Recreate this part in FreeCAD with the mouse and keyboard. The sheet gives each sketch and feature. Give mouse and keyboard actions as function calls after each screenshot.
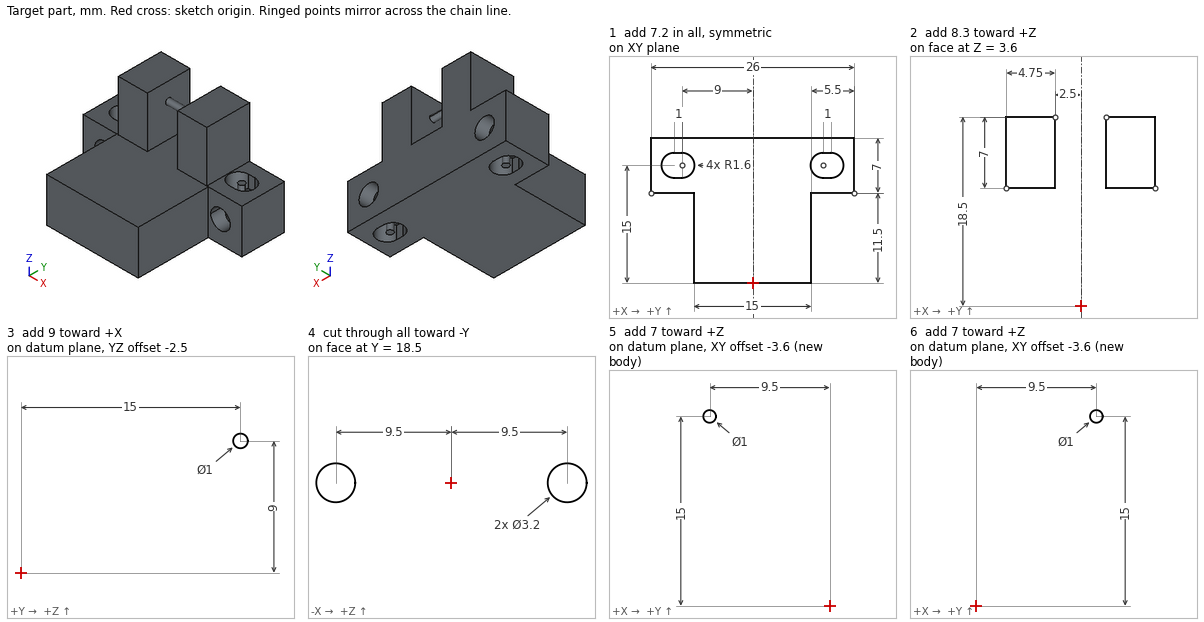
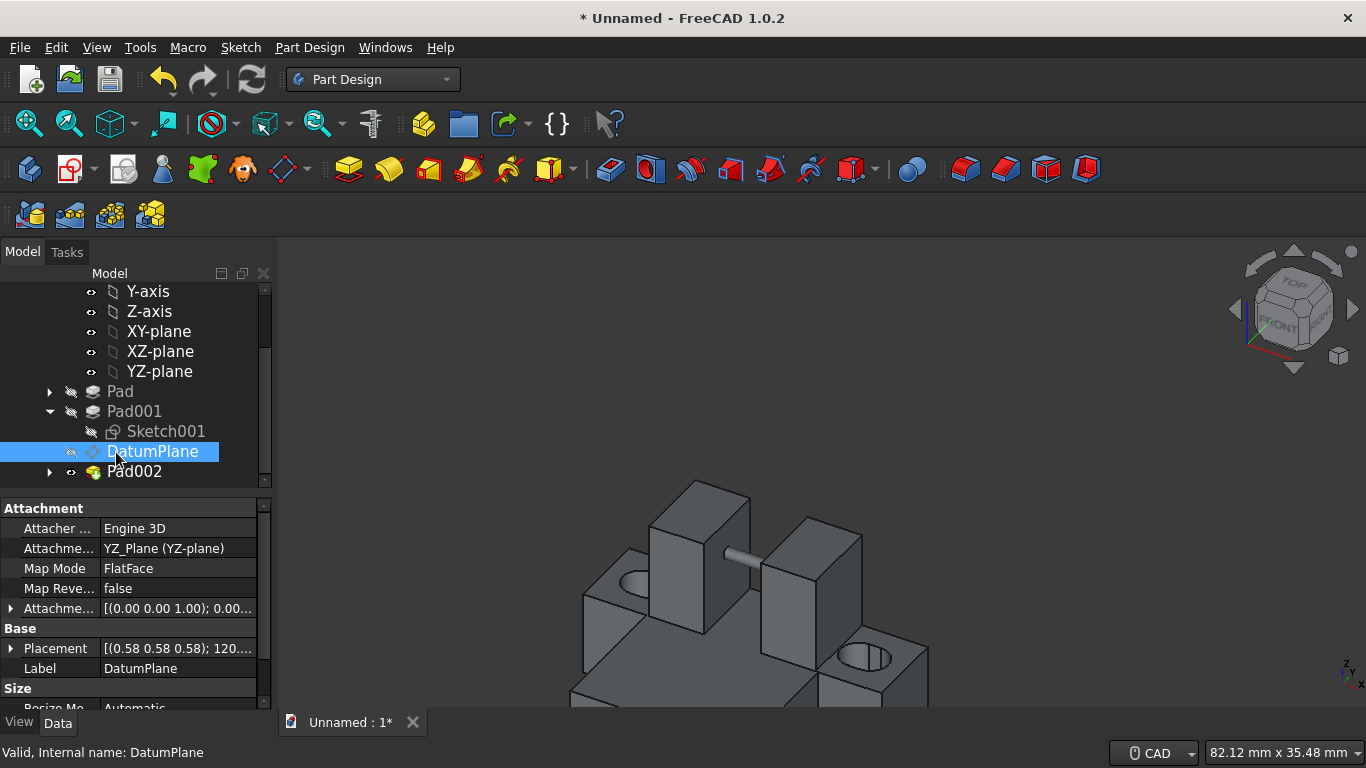
click(30, 124)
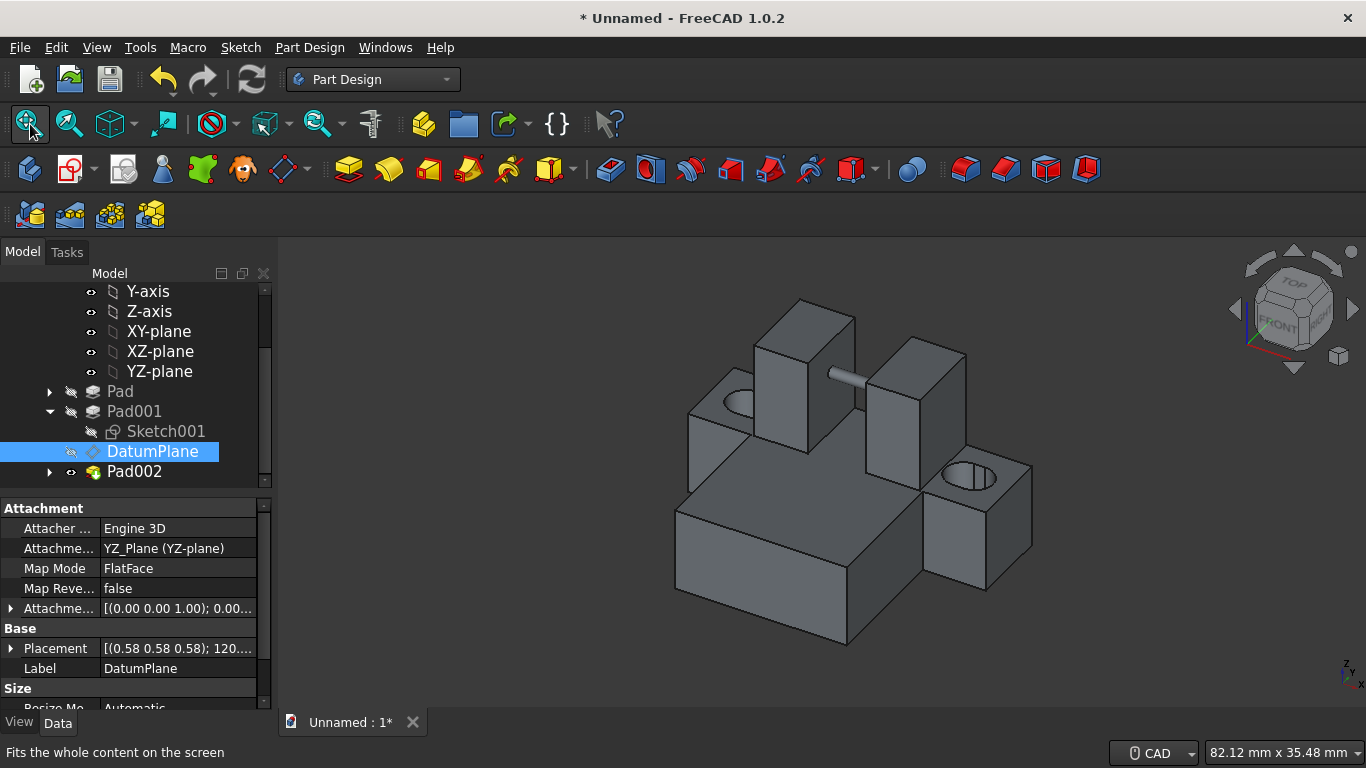
key(4)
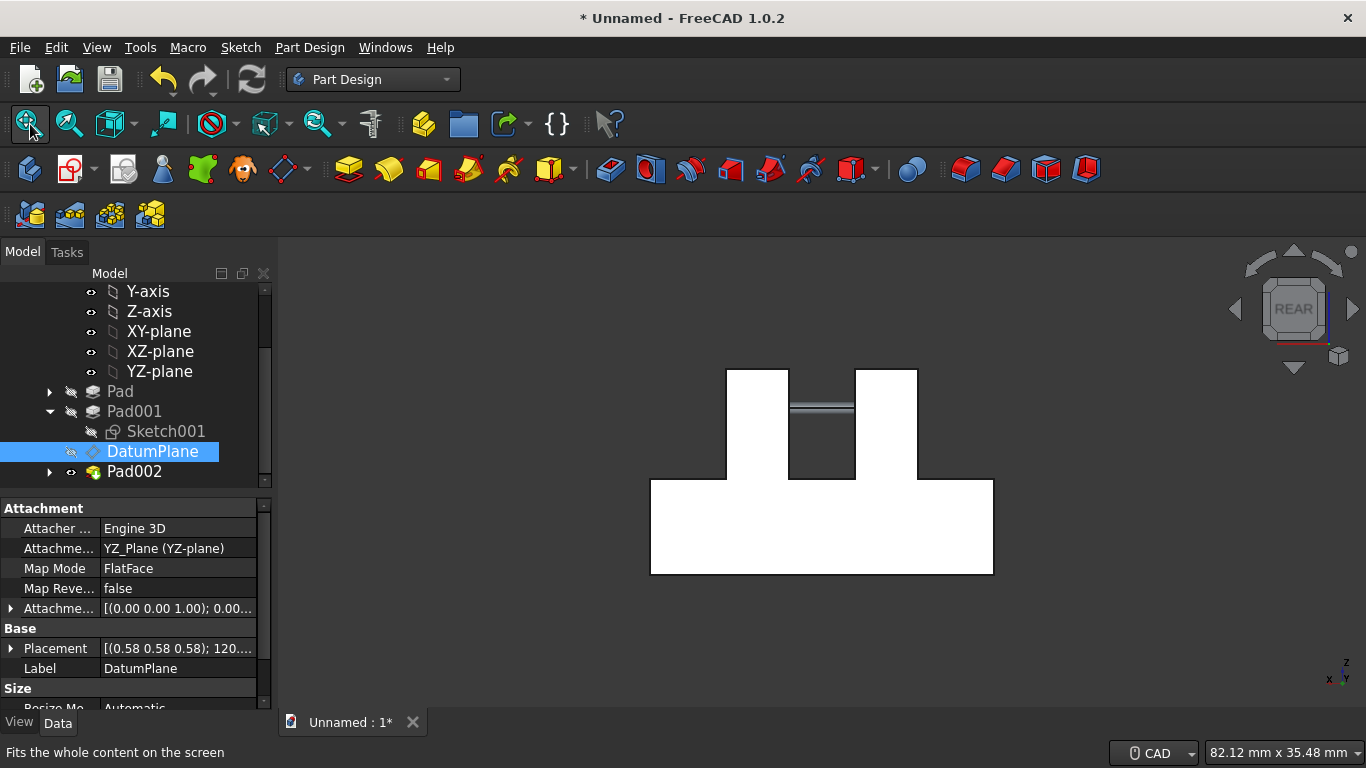
key(v)
key(f)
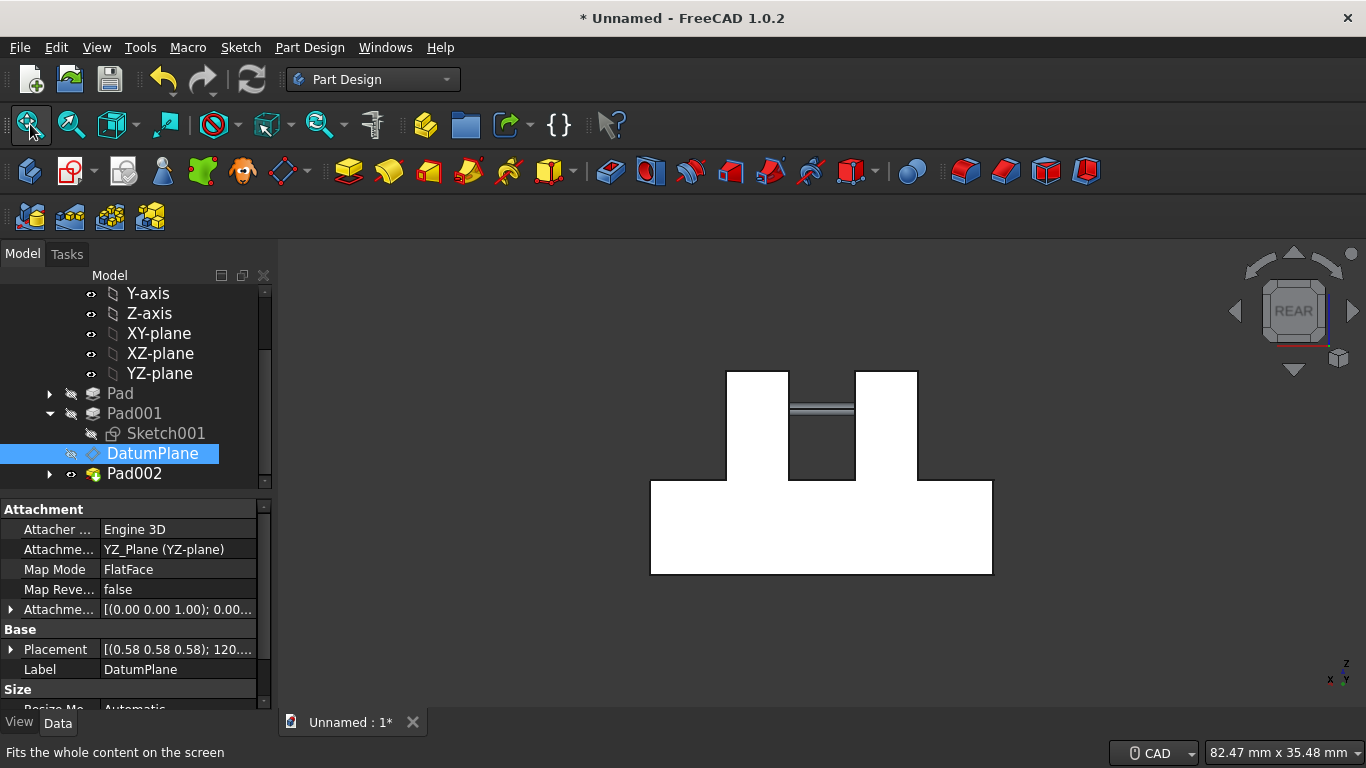
click(724, 530)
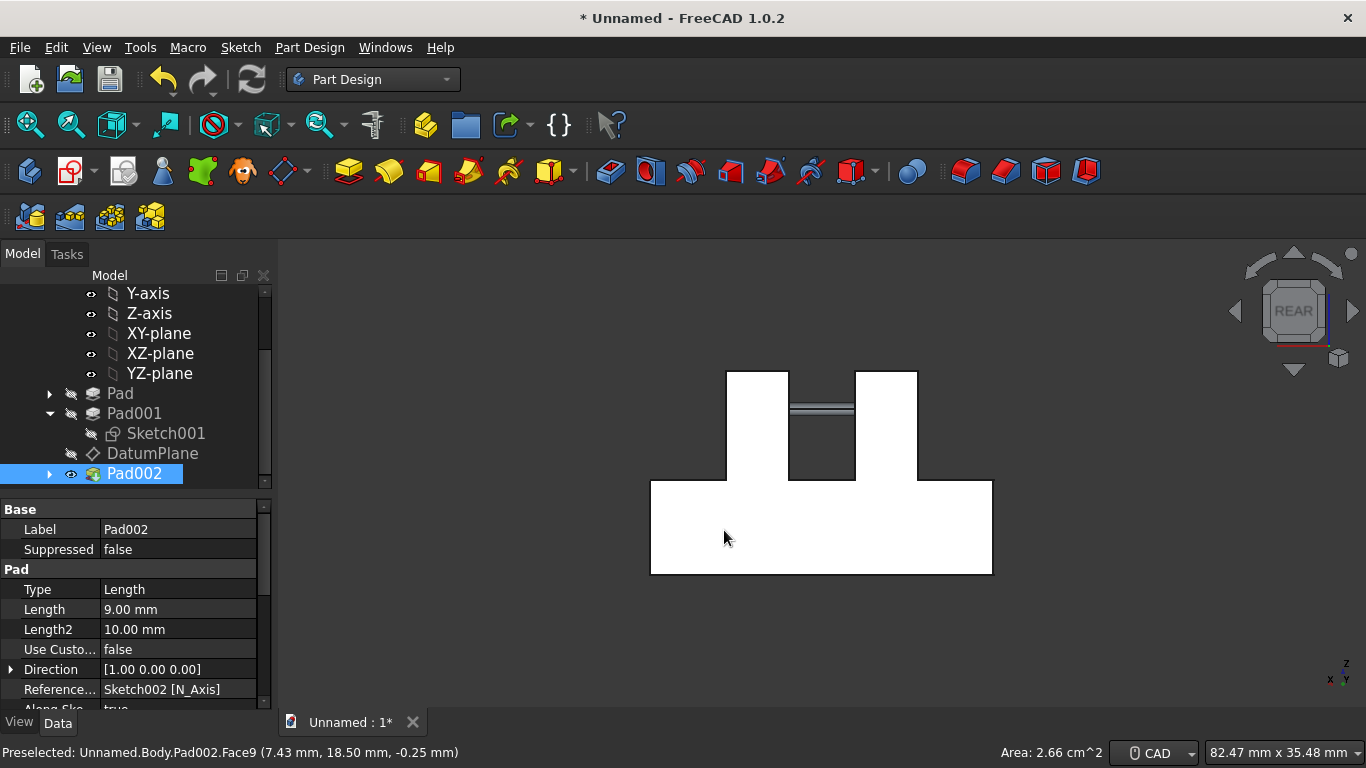
click(70, 172)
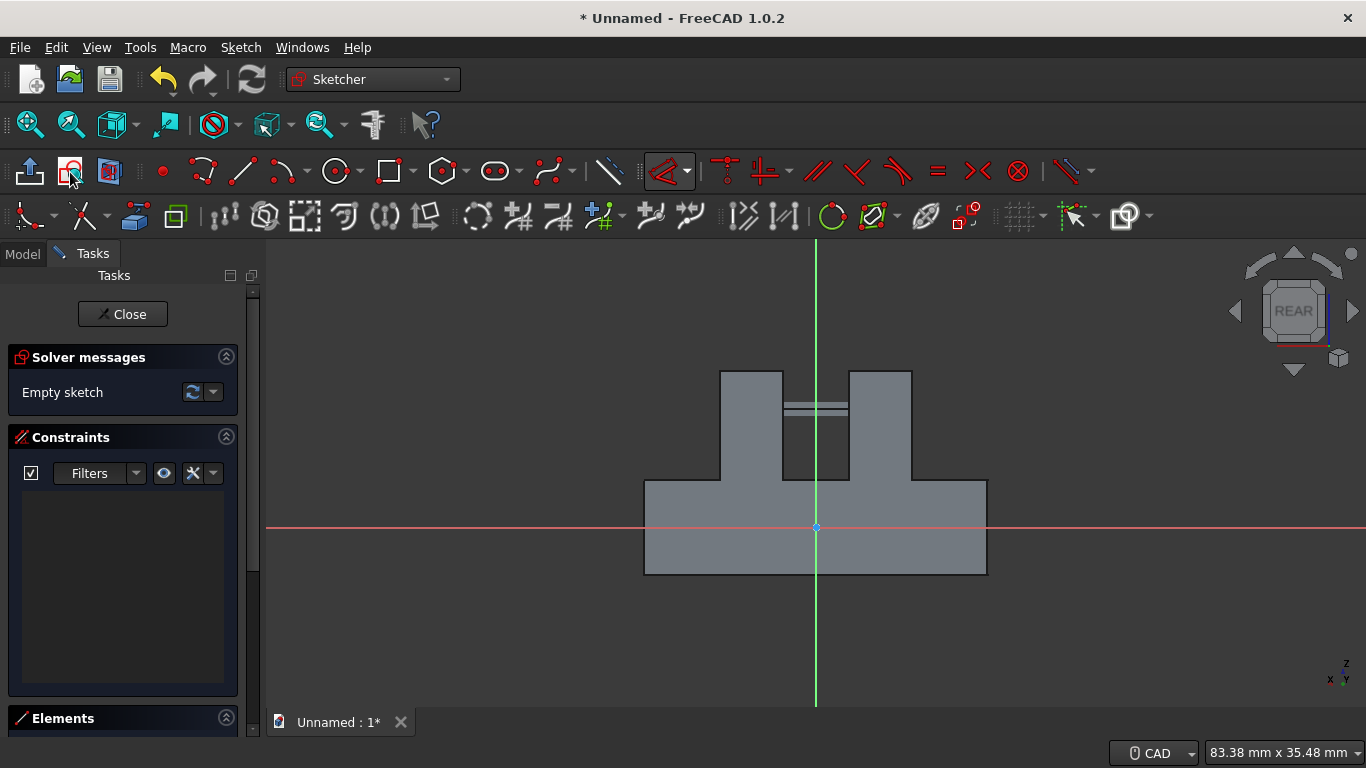
scroll(872, 572, up, 4)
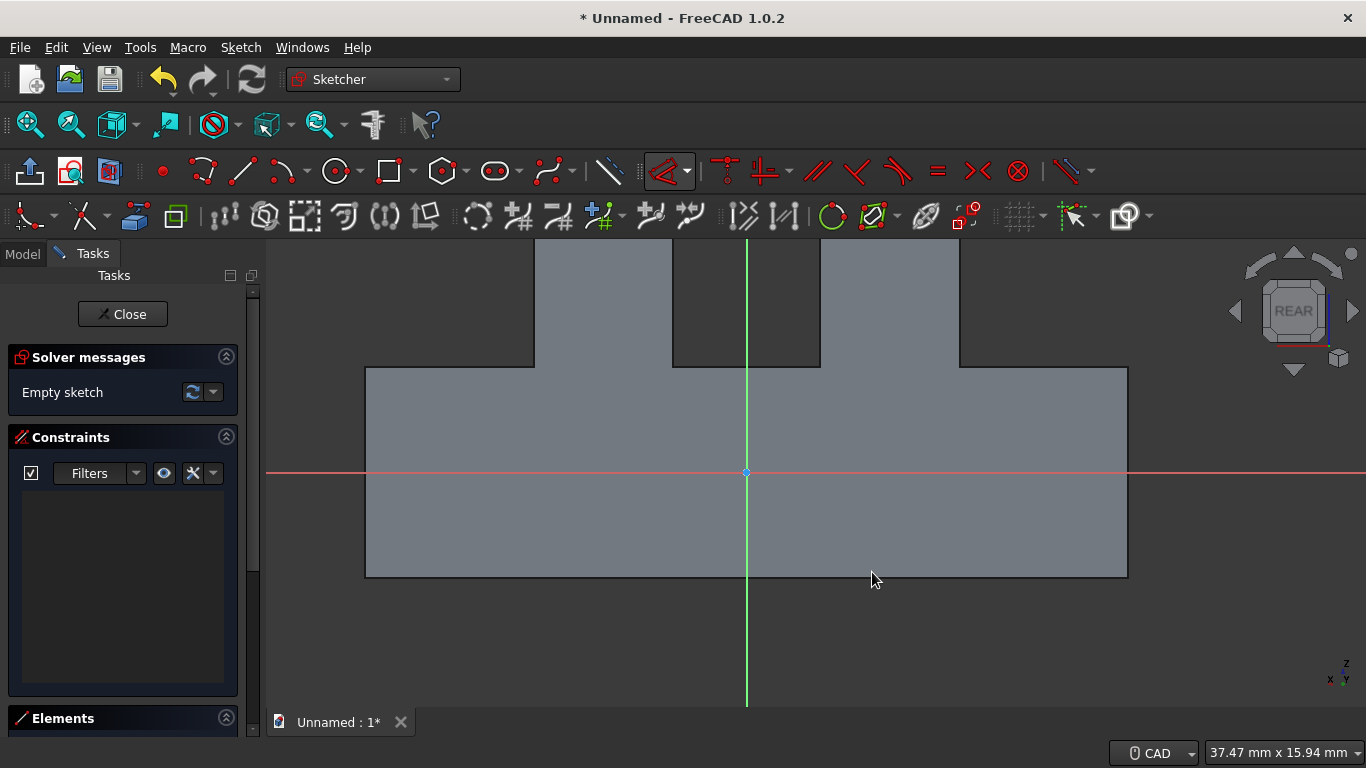
key(g)
key(c)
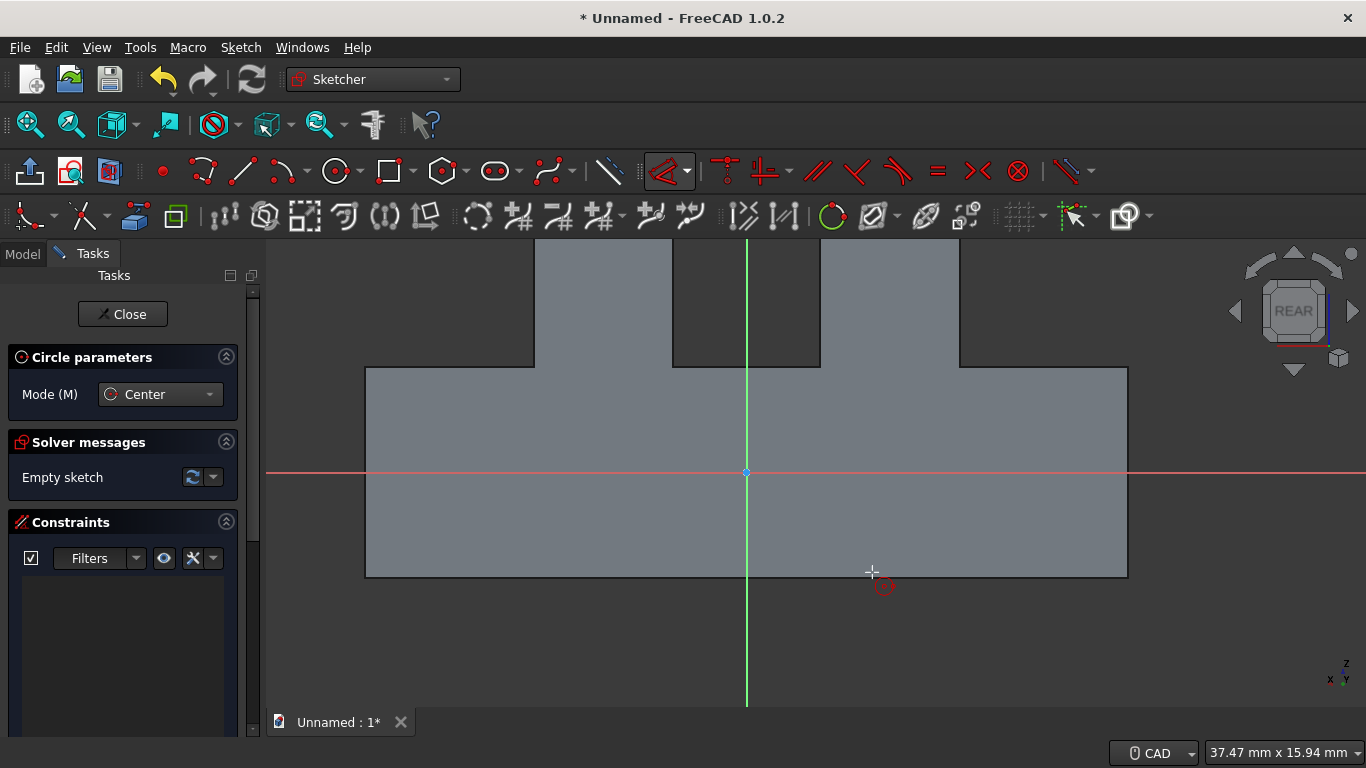
click(1026, 473)
click(1059, 439)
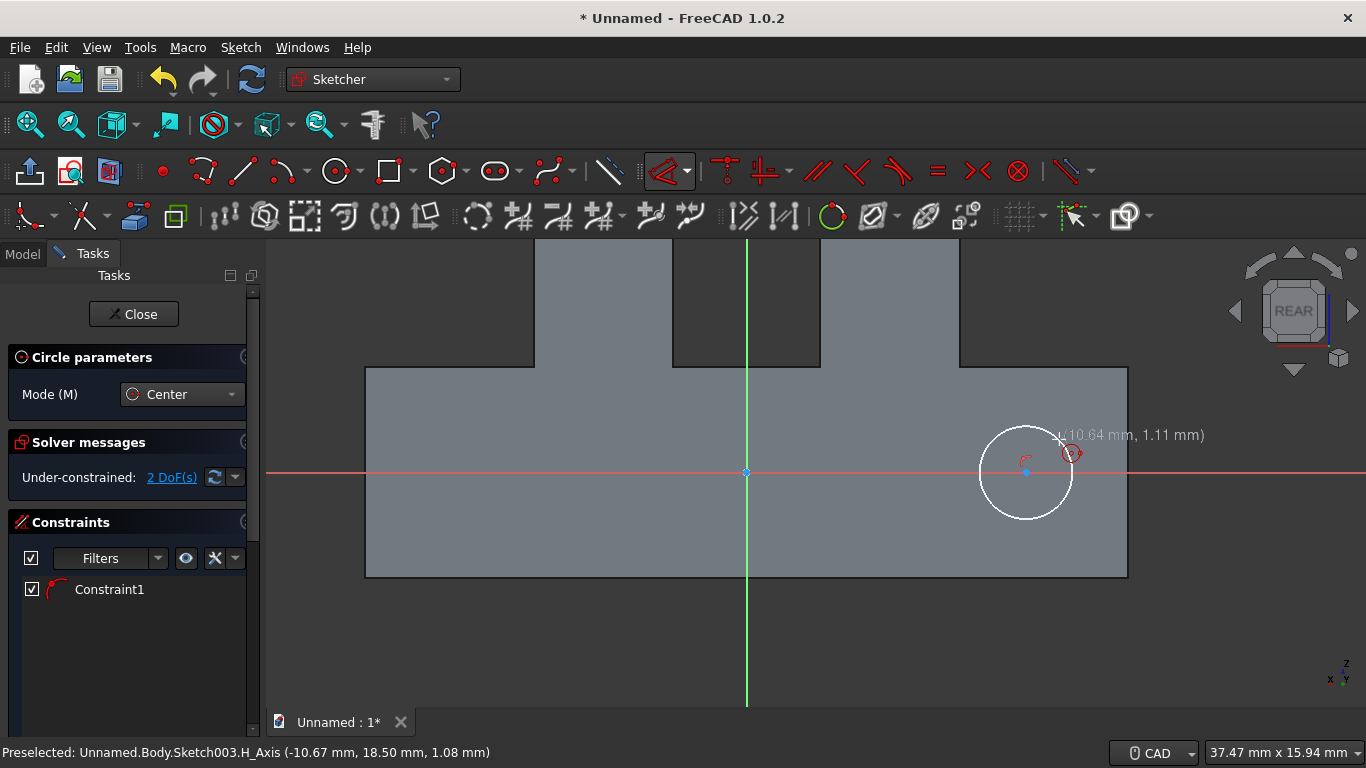
click(468, 473)
click(501, 439)
key(Escape)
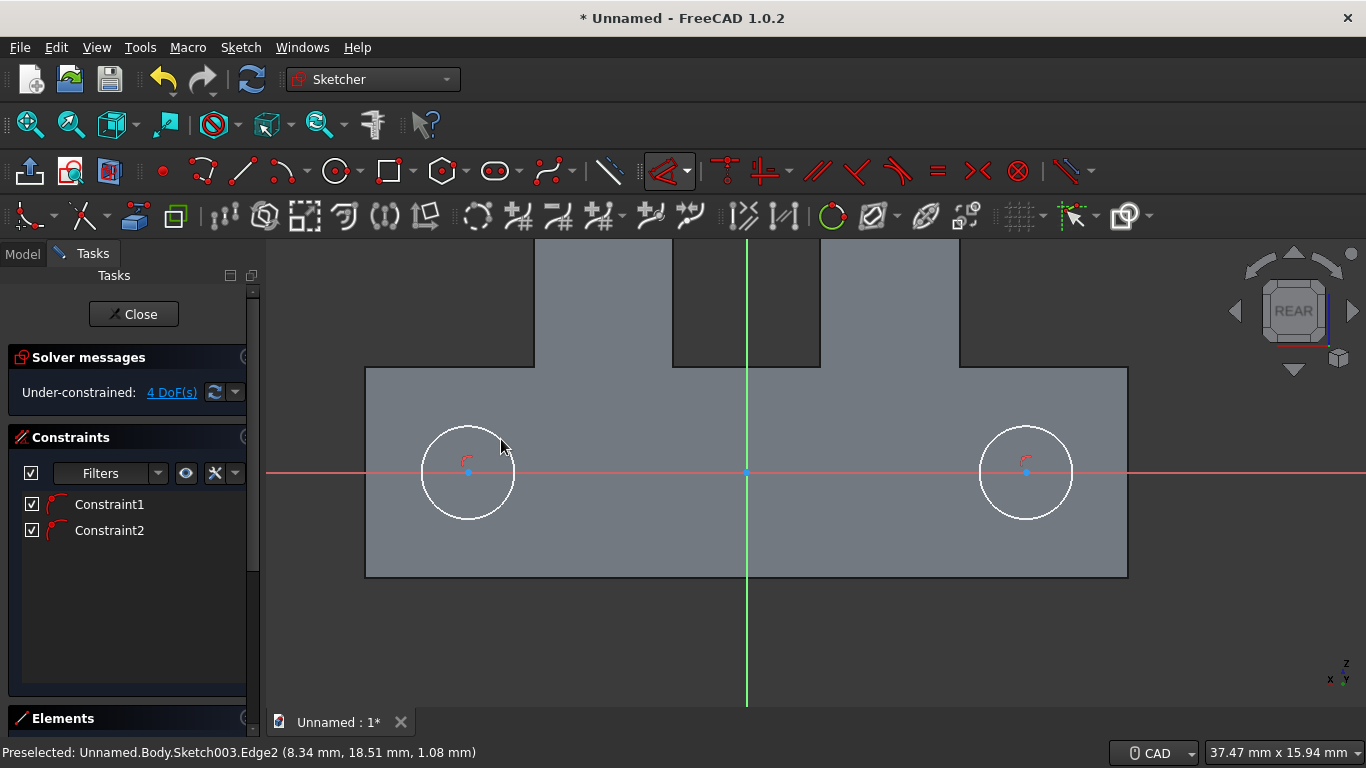
click(1059, 440)